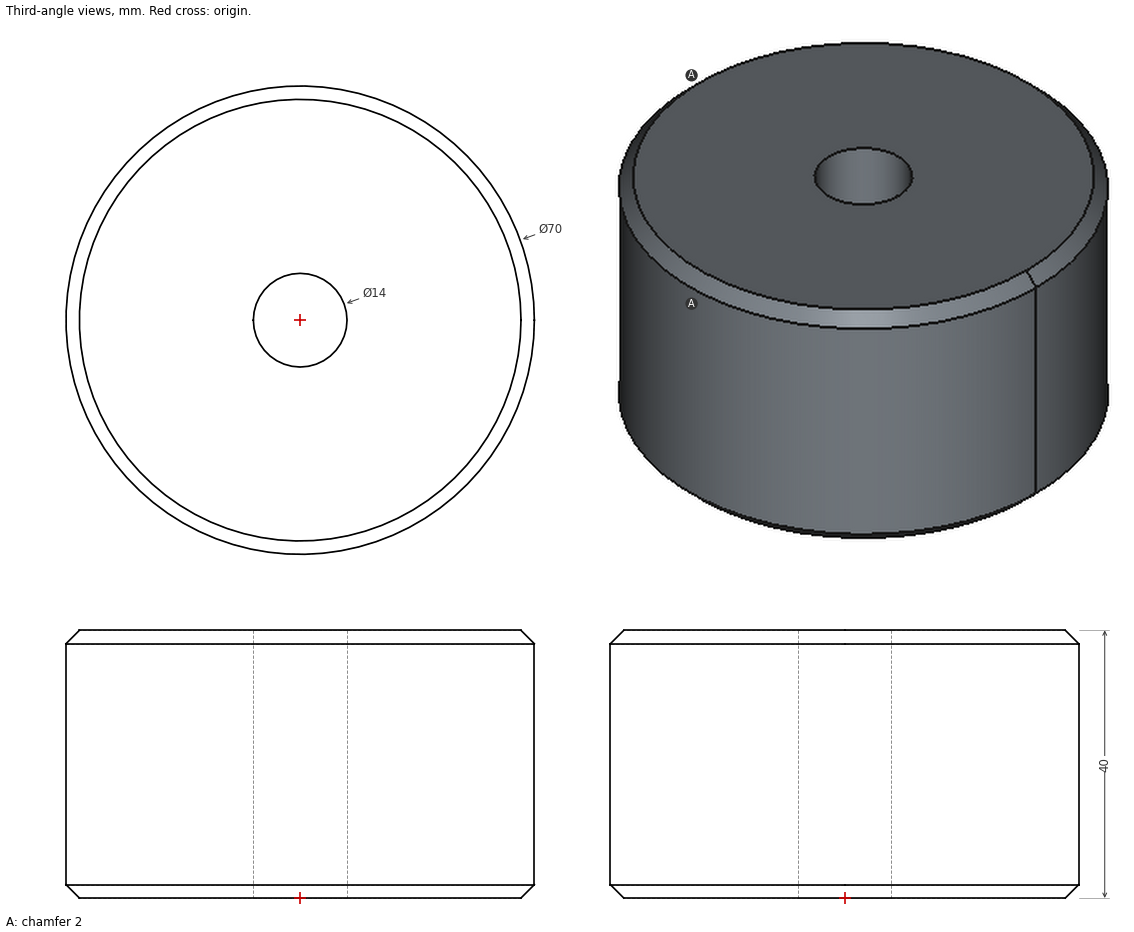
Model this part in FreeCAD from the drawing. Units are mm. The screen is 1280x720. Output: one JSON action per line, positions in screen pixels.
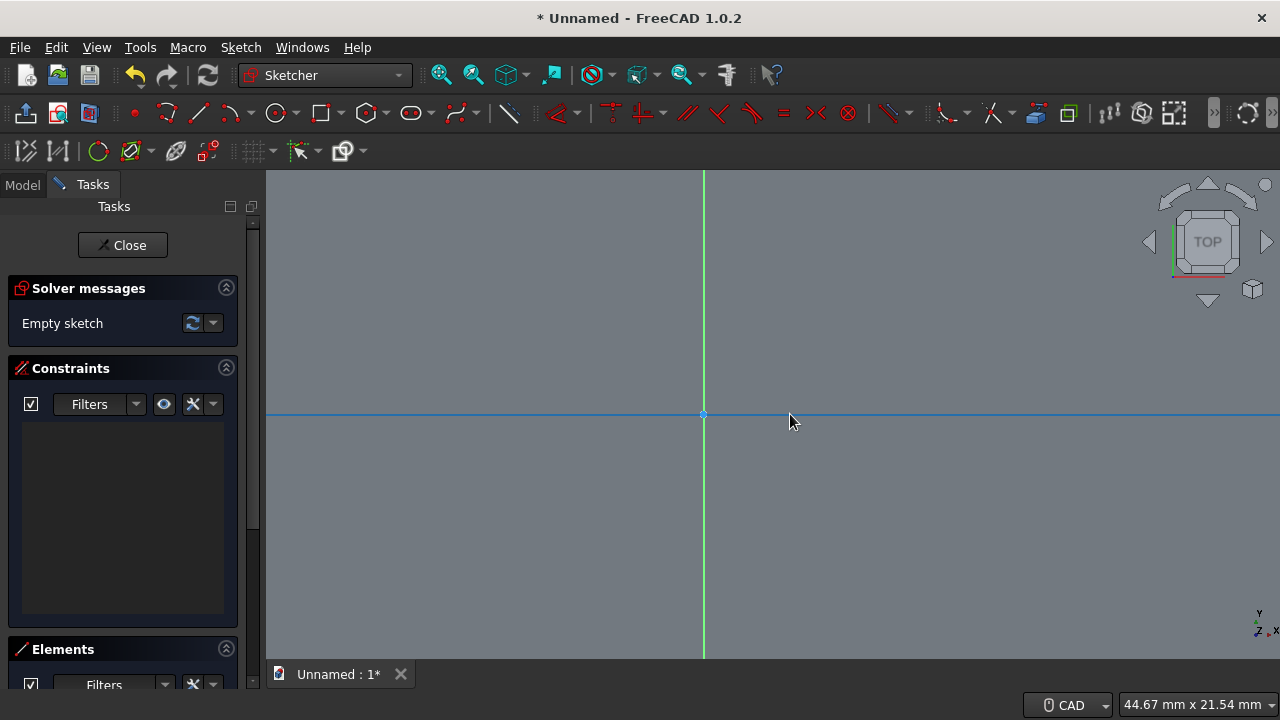
{"action": "key", "text": "g c"}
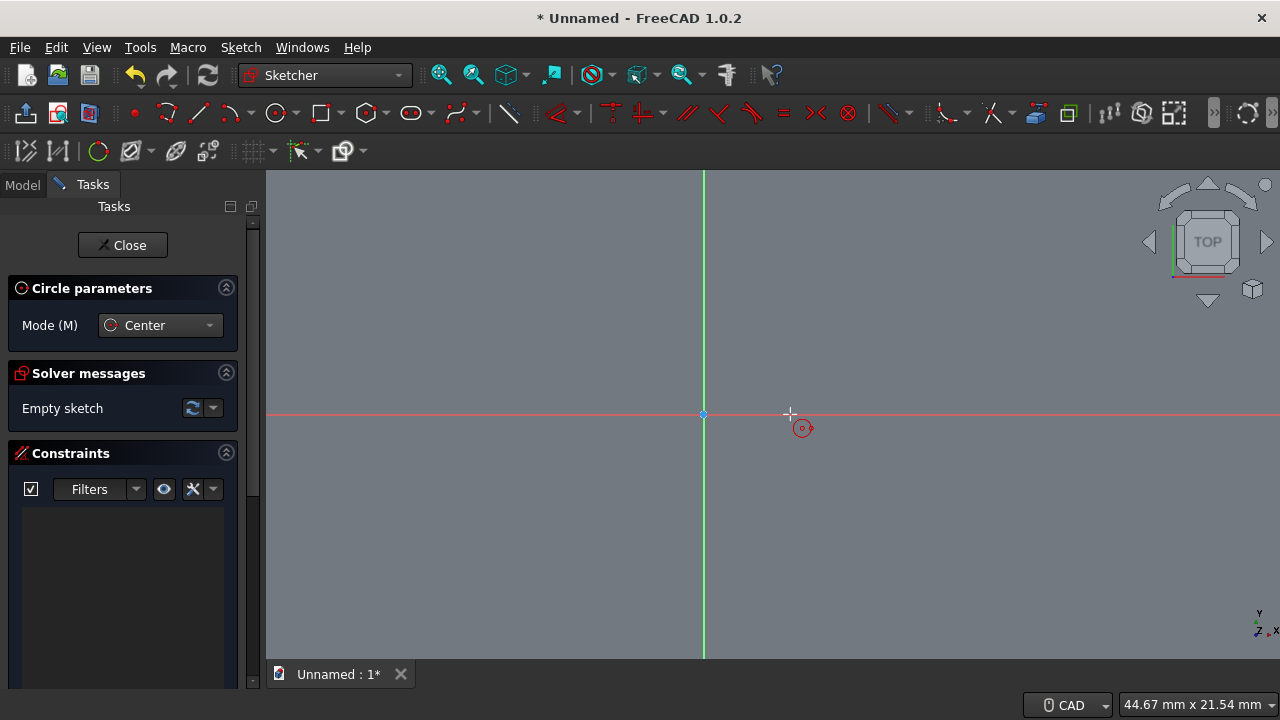
{"action": "left_click", "coordinate": [704, 414]}
{"action": "left_click", "coordinate": [816, 302]}
{"action": "key", "text": "Escape"}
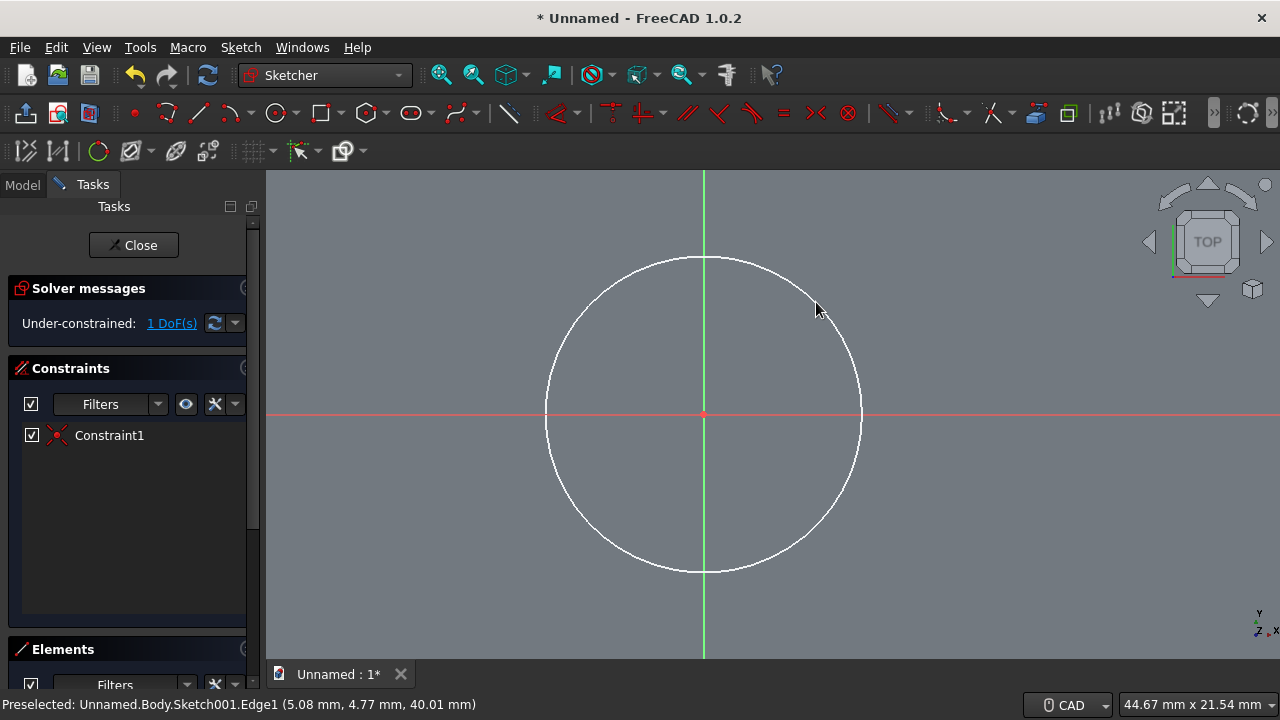
{"action": "left_click", "coordinate": [556, 114]}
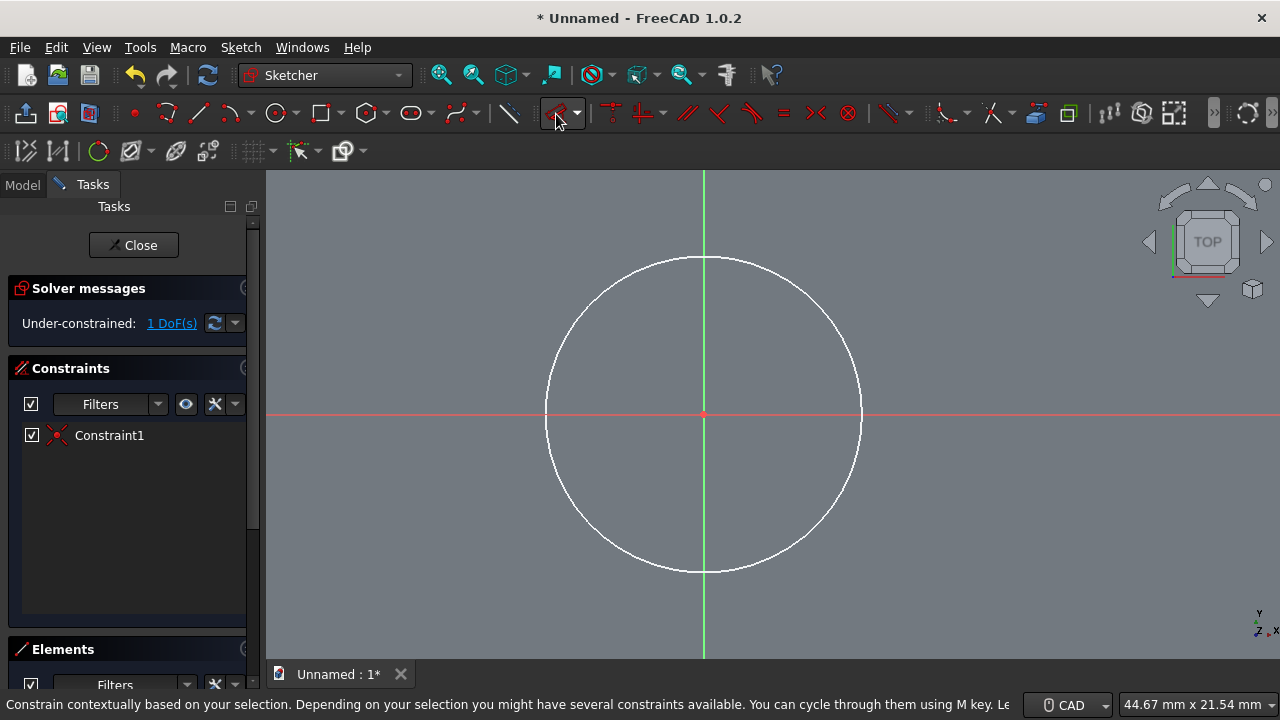
{"action": "left_click", "coordinate": [815, 302]}
{"action": "left_click", "coordinate": [838, 279]}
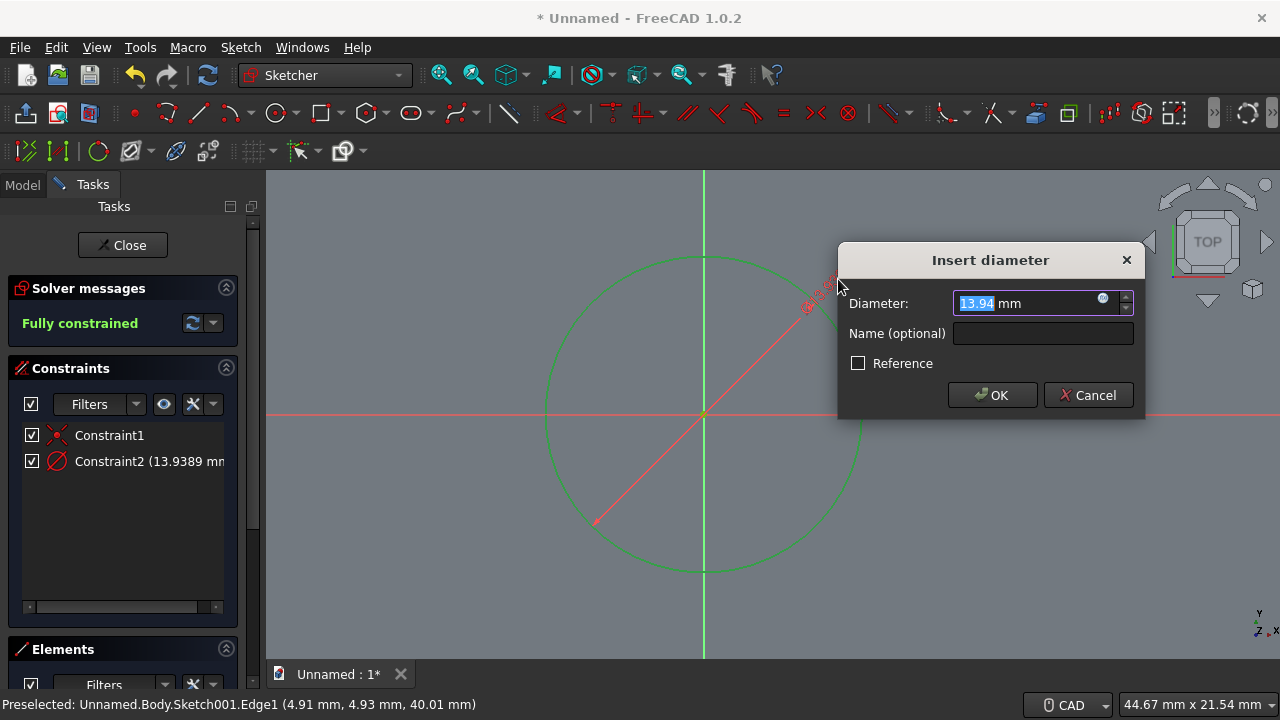
{"action": "type", "text": "14"}
{"action": "key", "text": "Return"}
{"action": "key", "text": "Escape"}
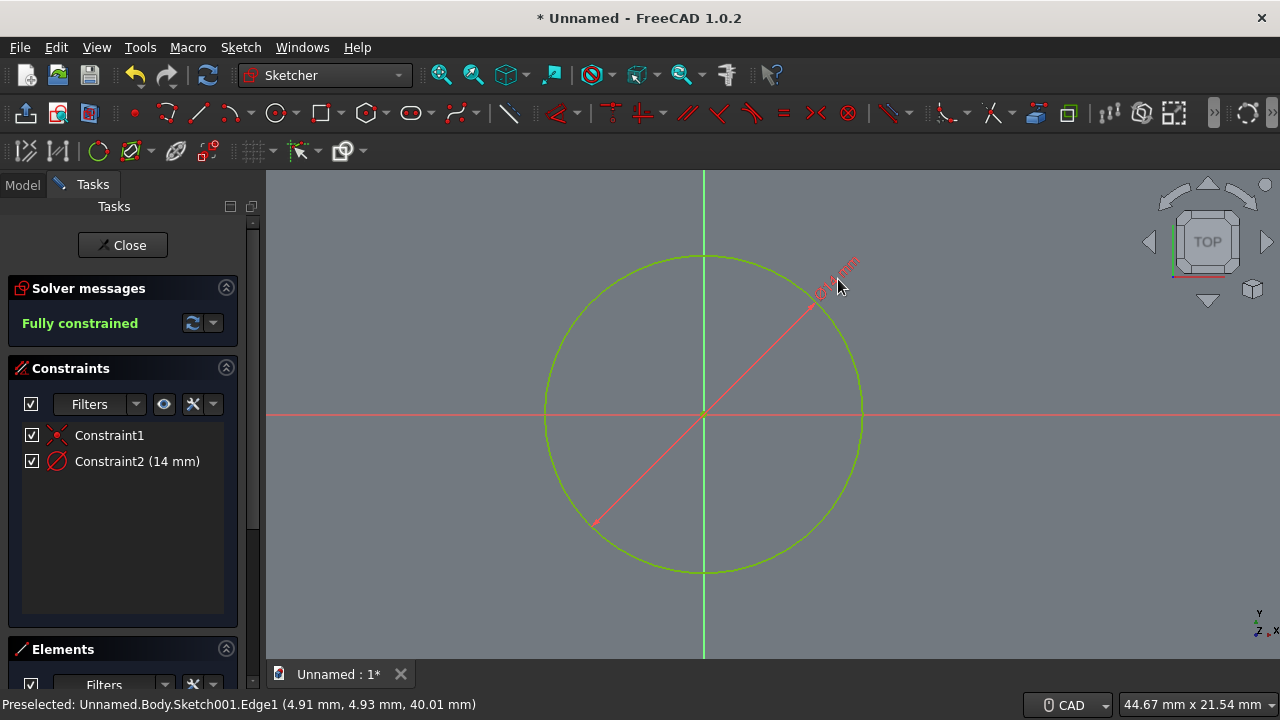
{"action": "left_click", "coordinate": [123, 245]}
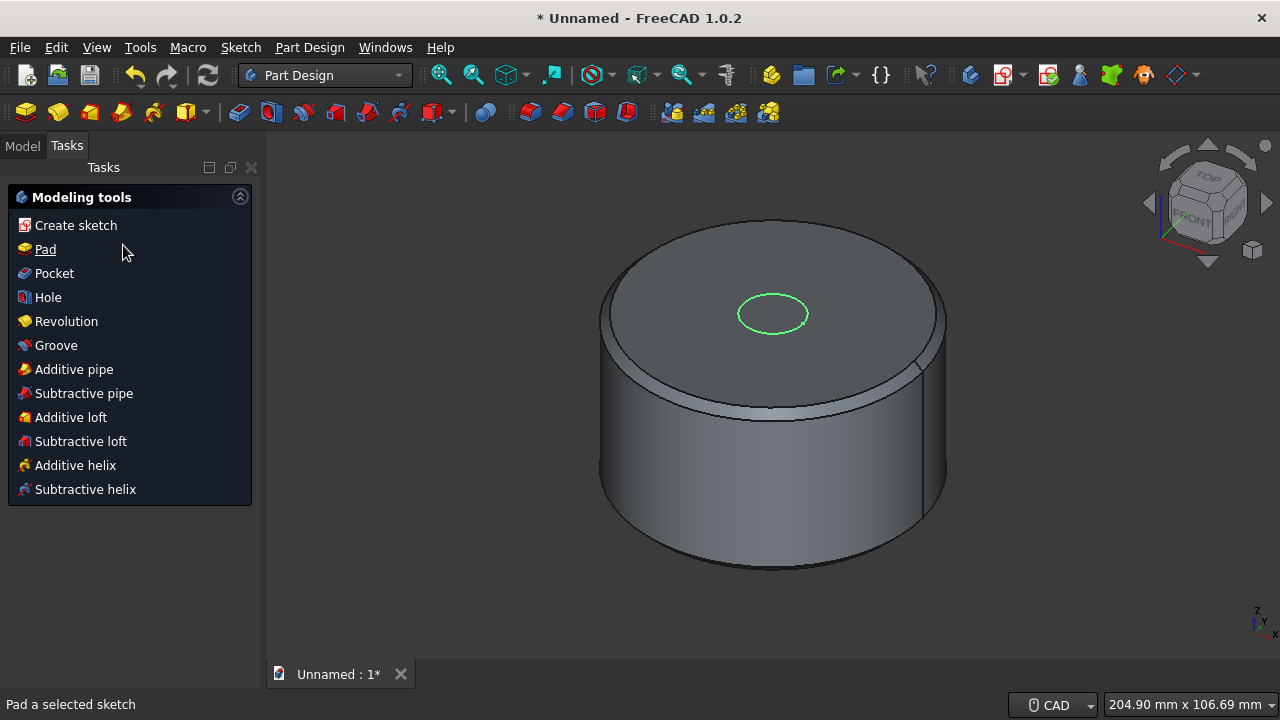
{"action": "left_click", "coordinate": [240, 112]}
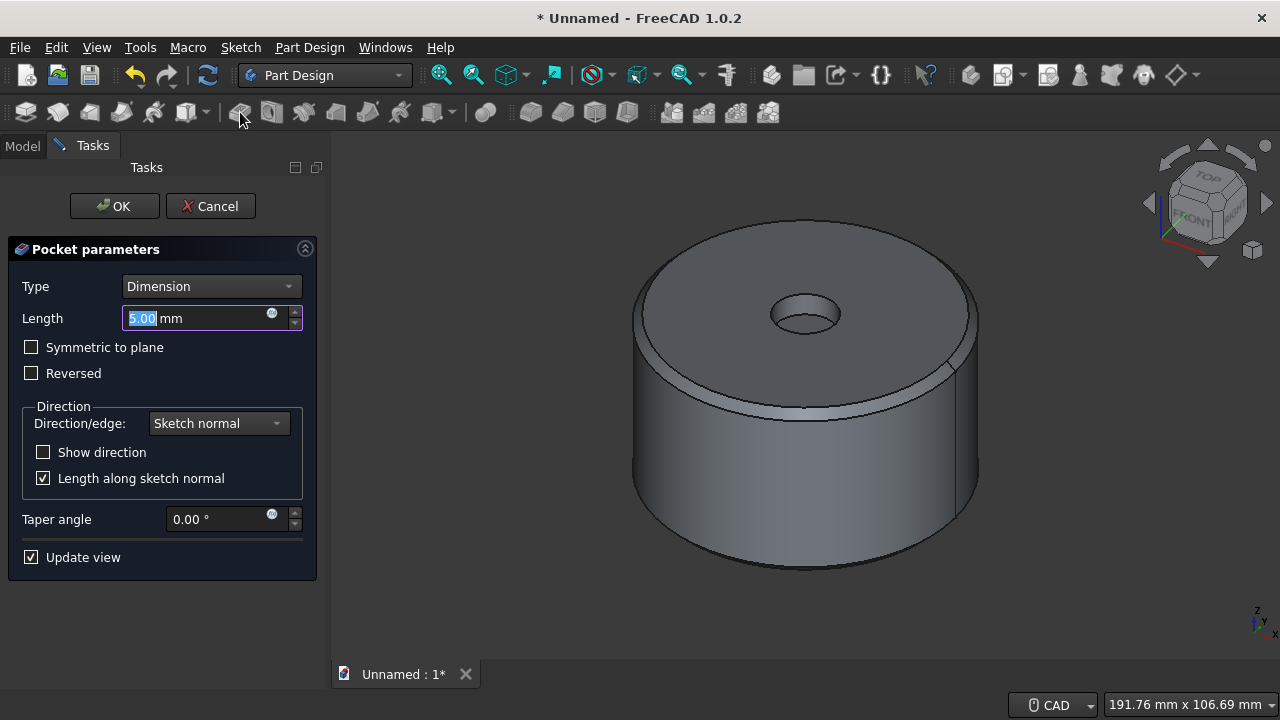
{"action": "left_click", "coordinate": [212, 286]}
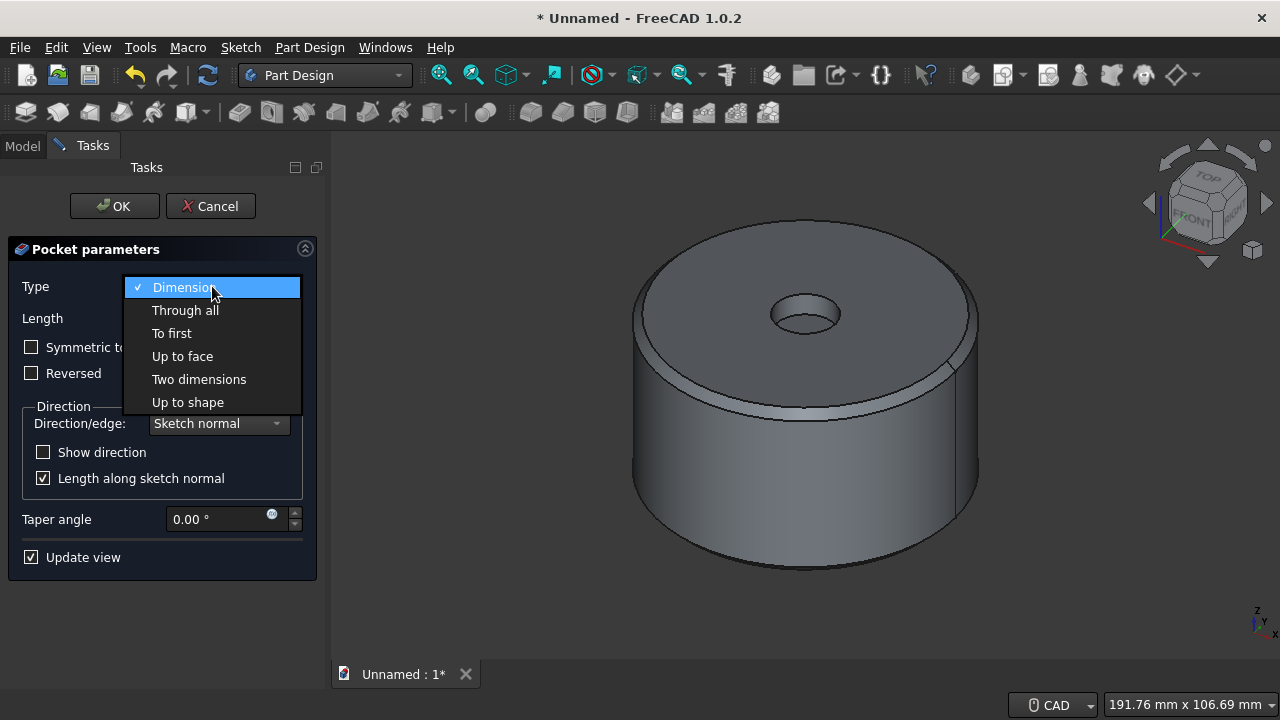
{"action": "left_click", "coordinate": [212, 310]}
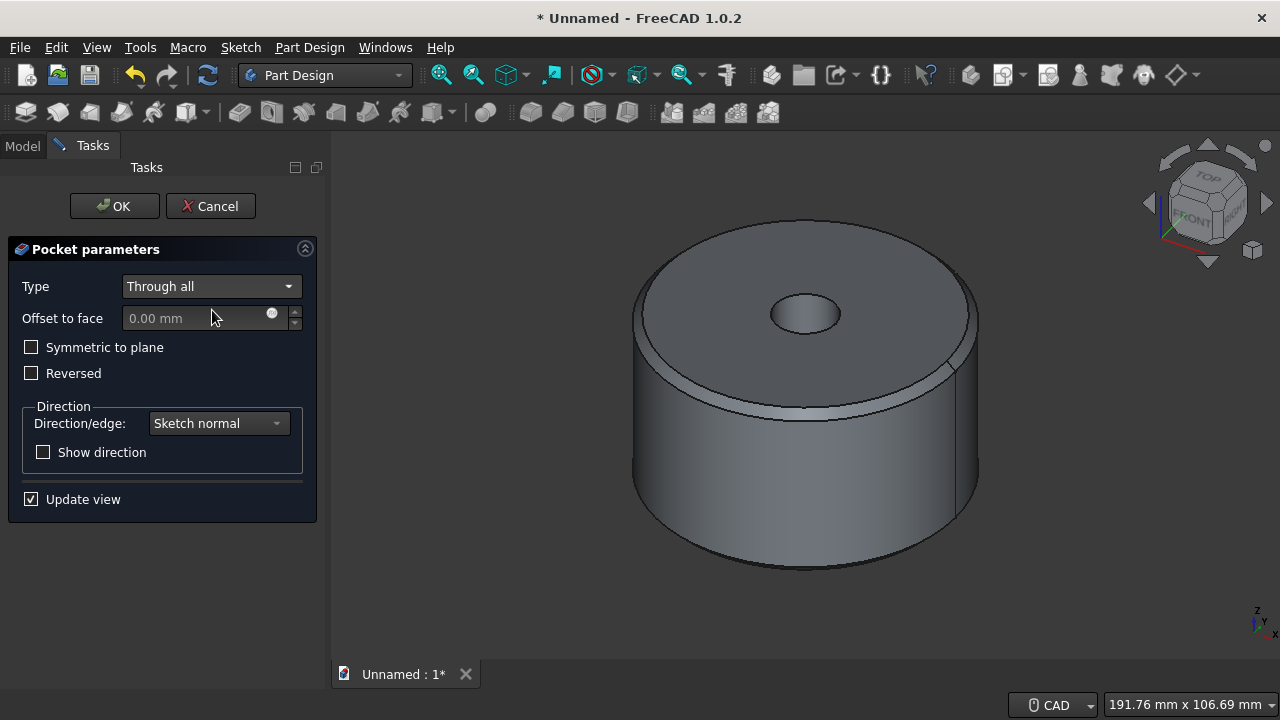
{"action": "left_click", "coordinate": [115, 206]}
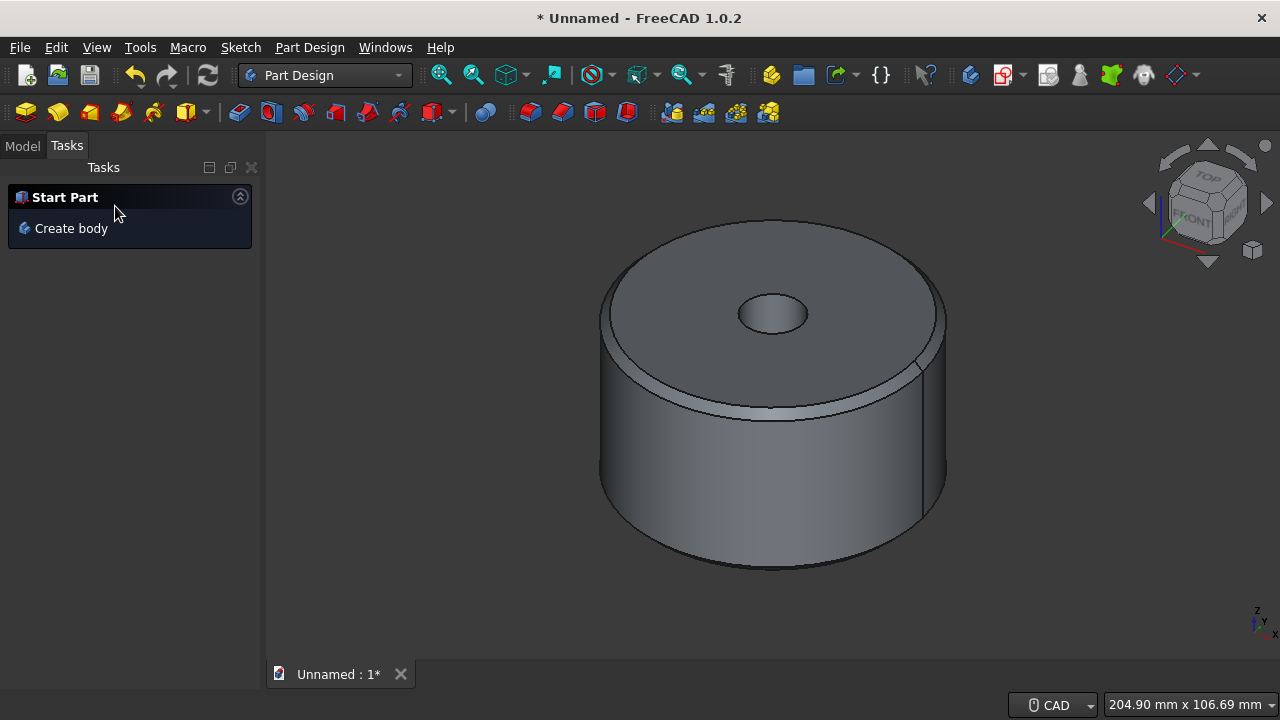
{"action": "key", "text": "0"}